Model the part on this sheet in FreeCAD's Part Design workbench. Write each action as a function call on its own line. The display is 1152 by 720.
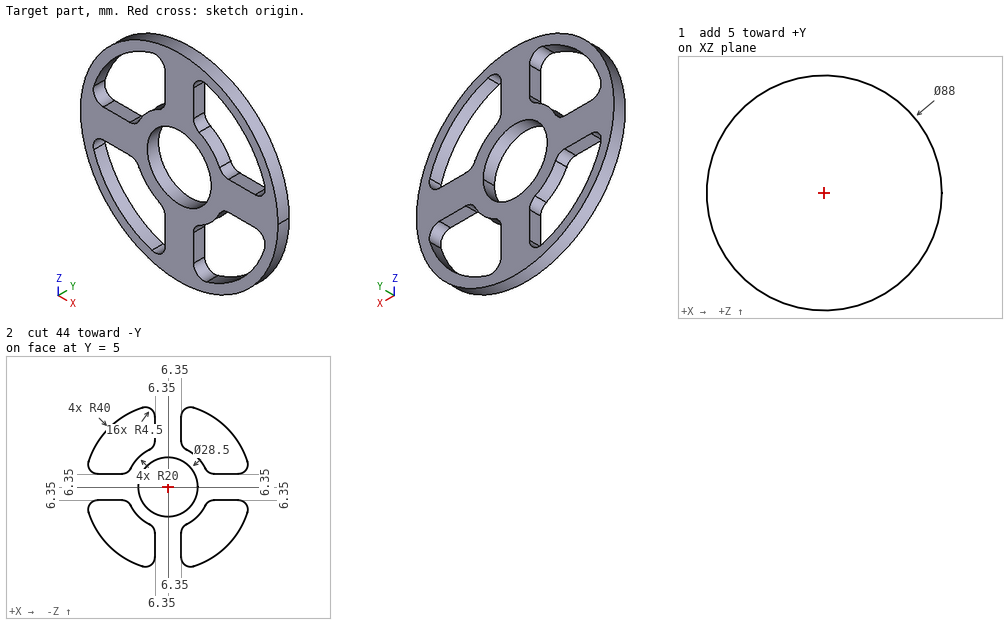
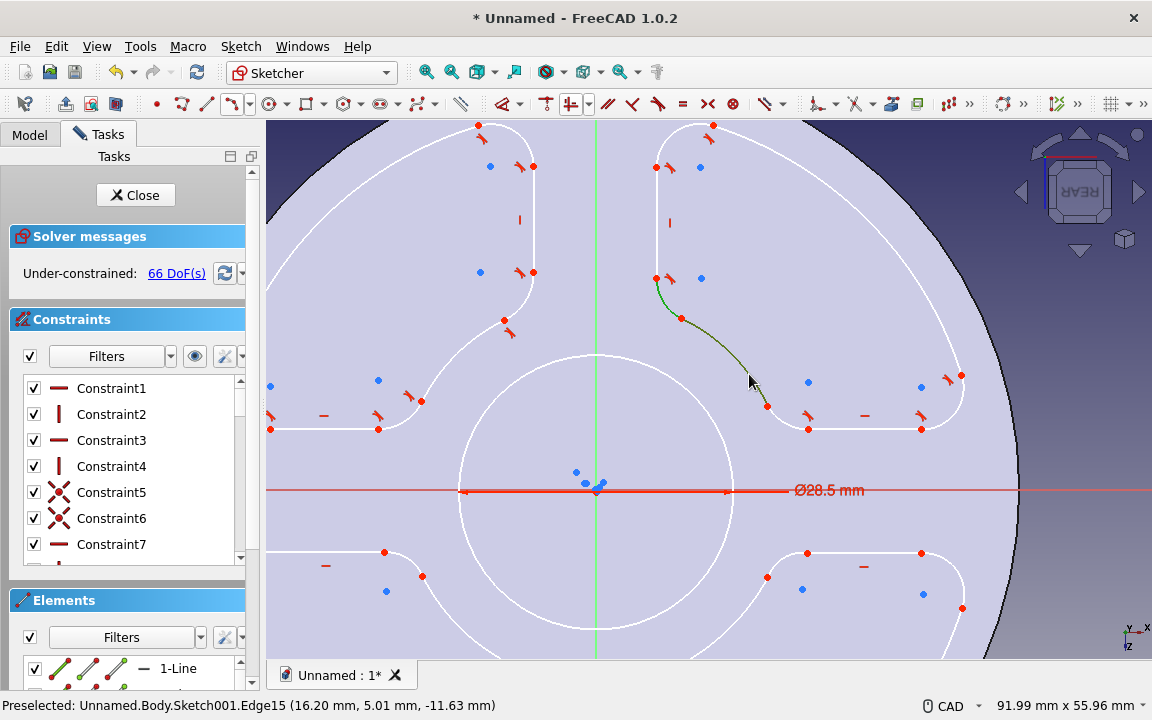
key(t)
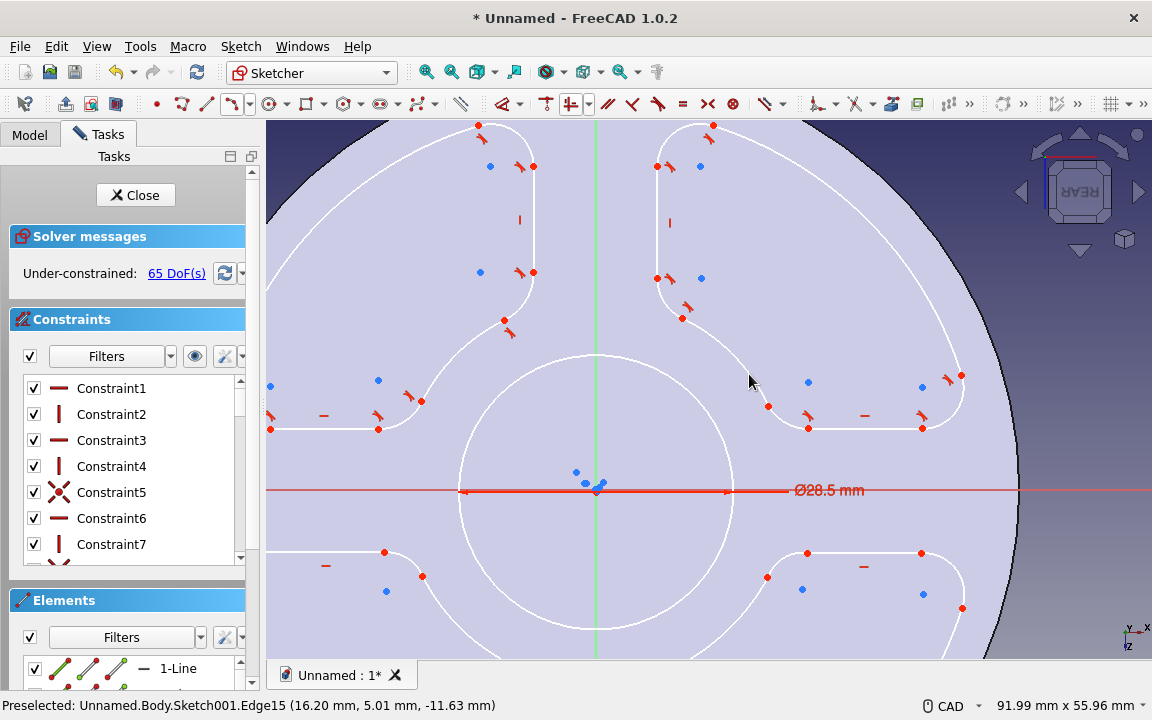
click(749, 374)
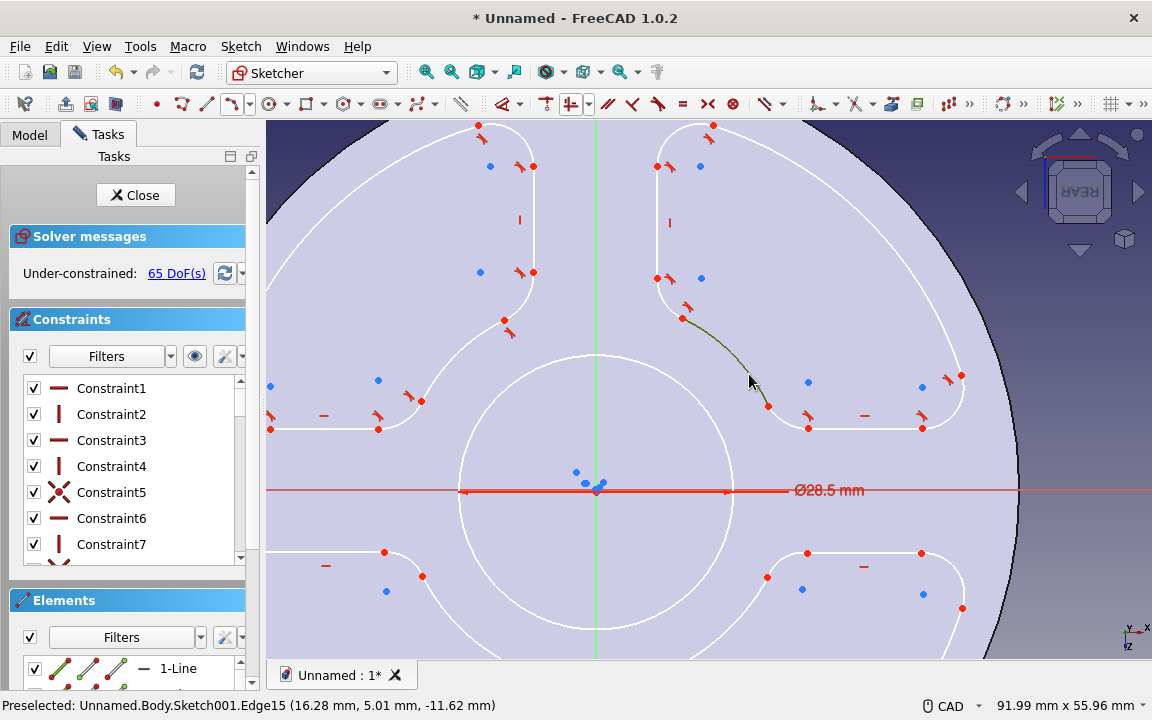
click(778, 417)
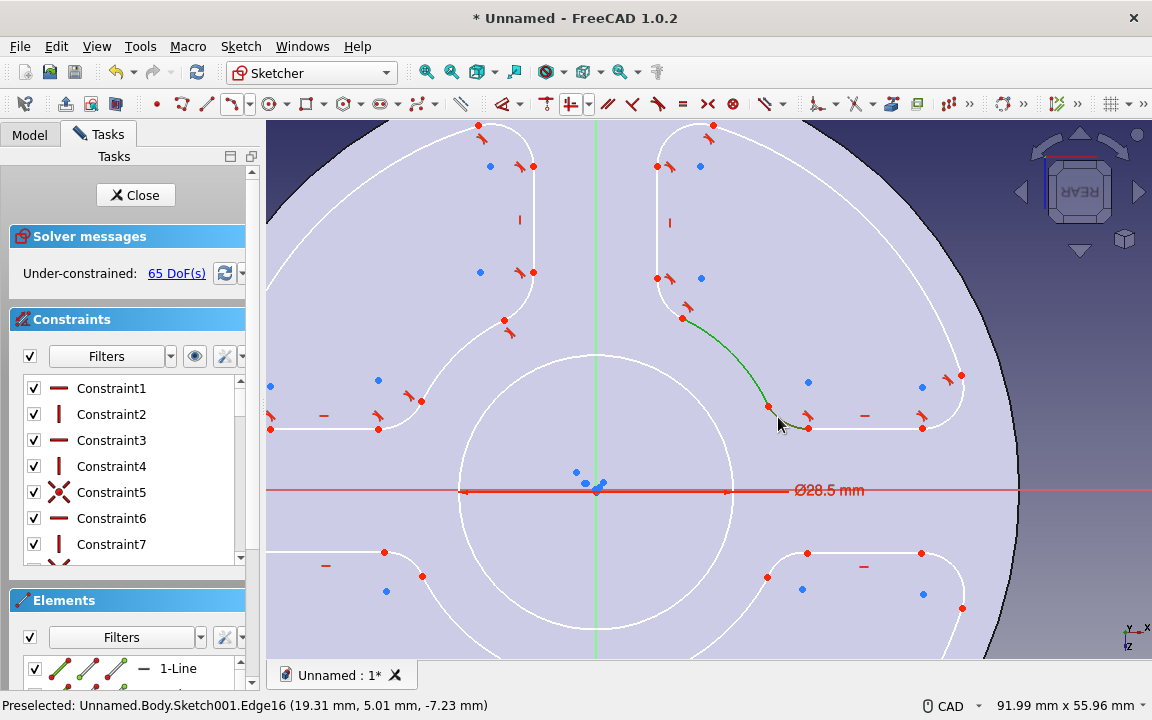
click(658, 104)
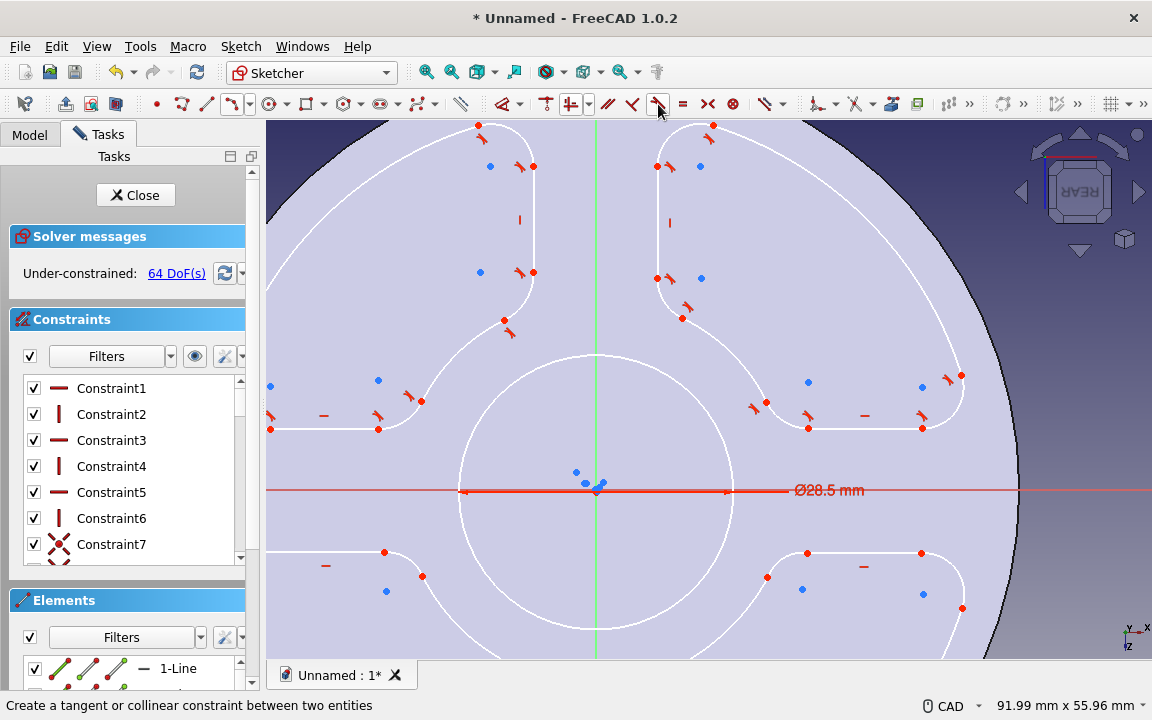
click(887, 553)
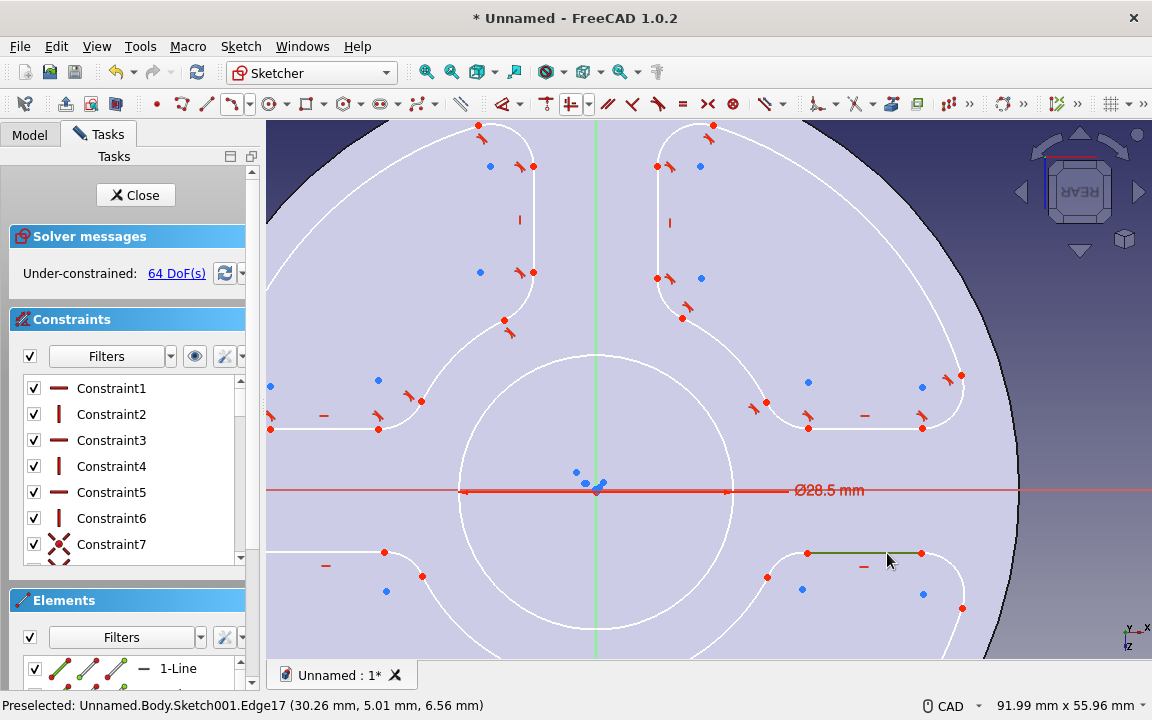
click(793, 554)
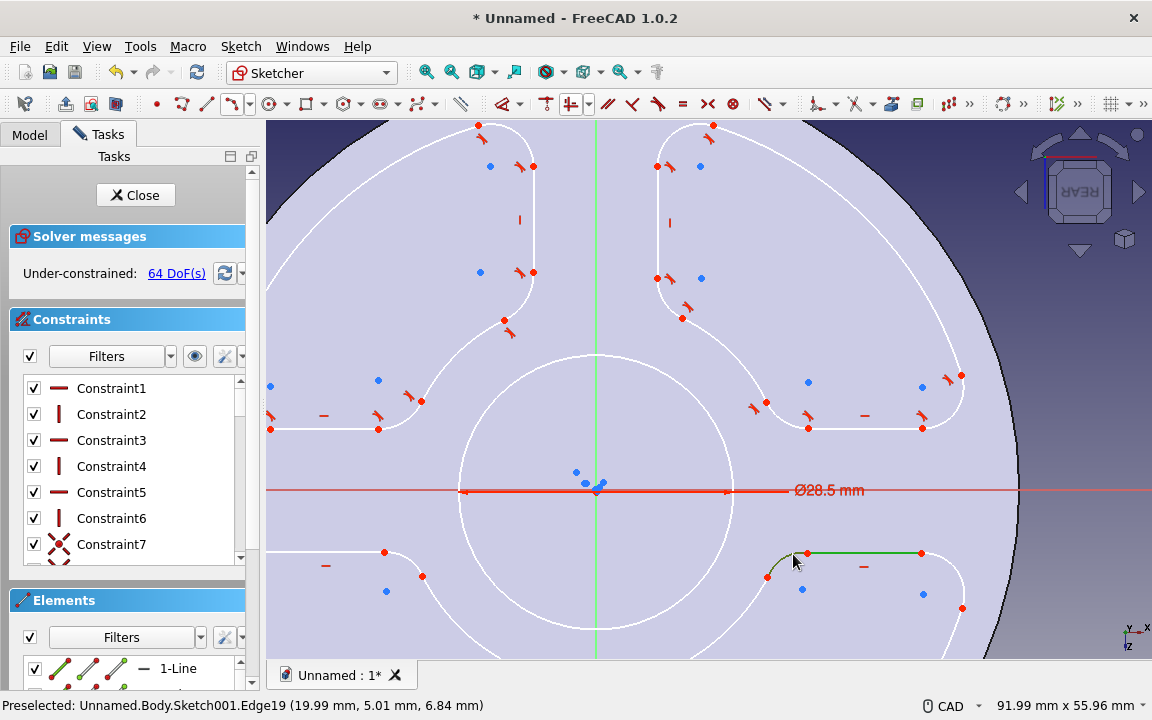
click(658, 104)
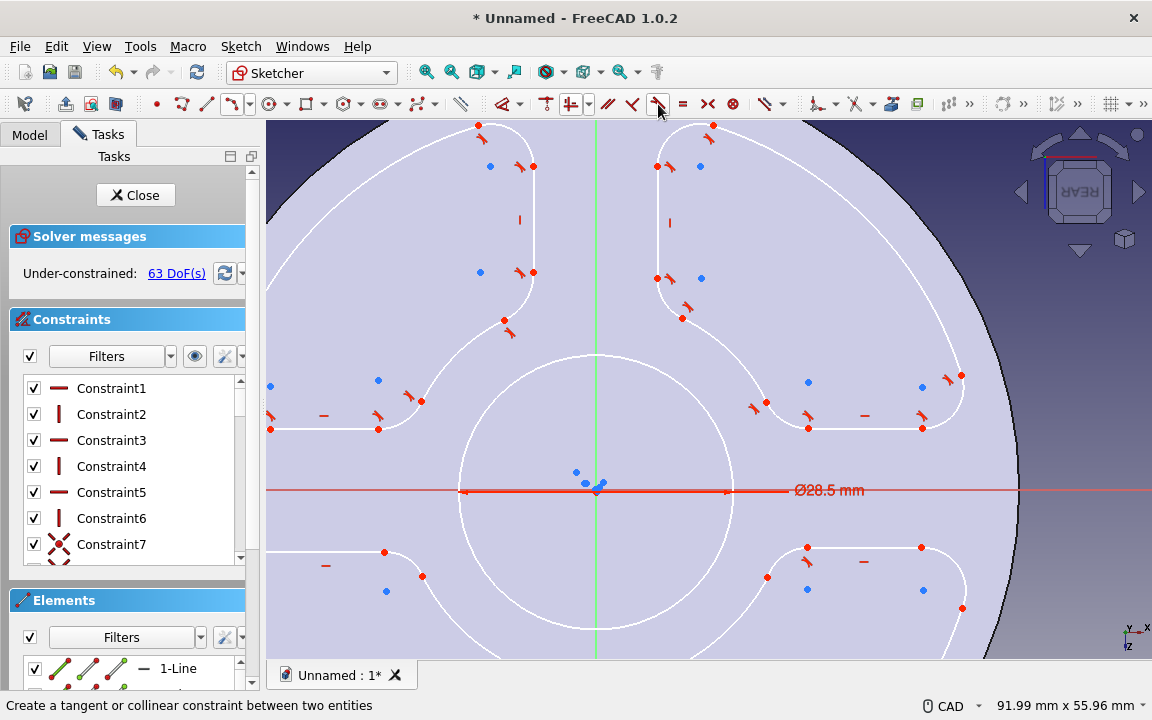
click(887, 548)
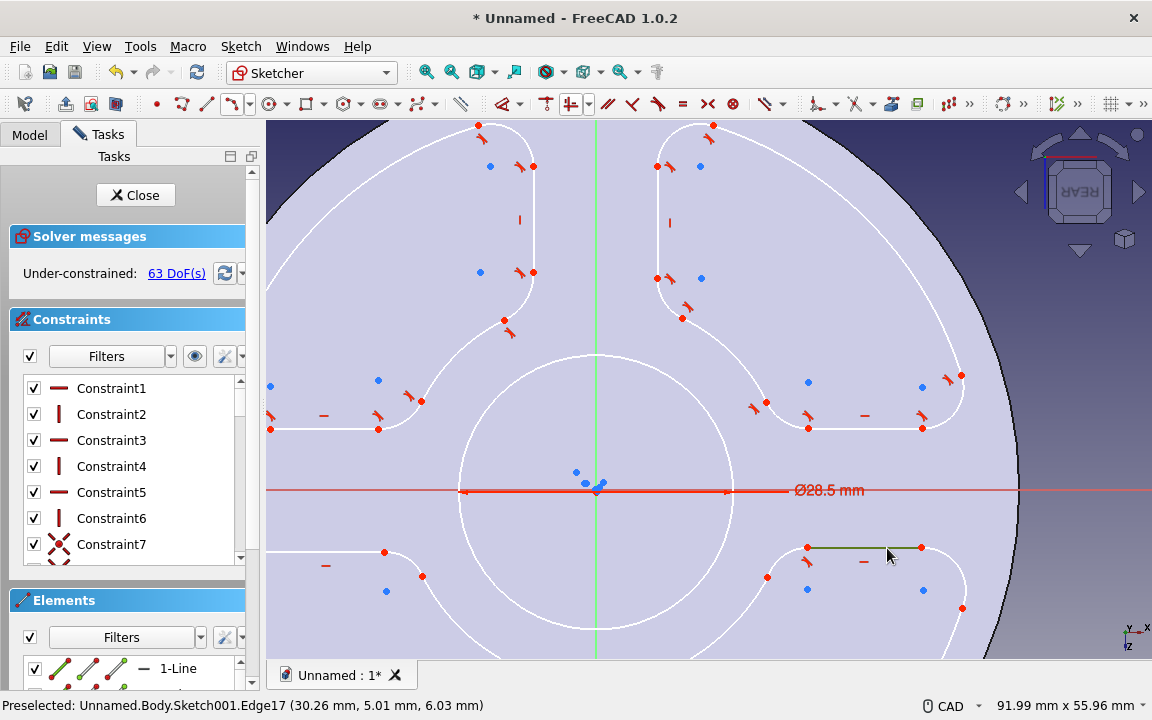
click(965, 583)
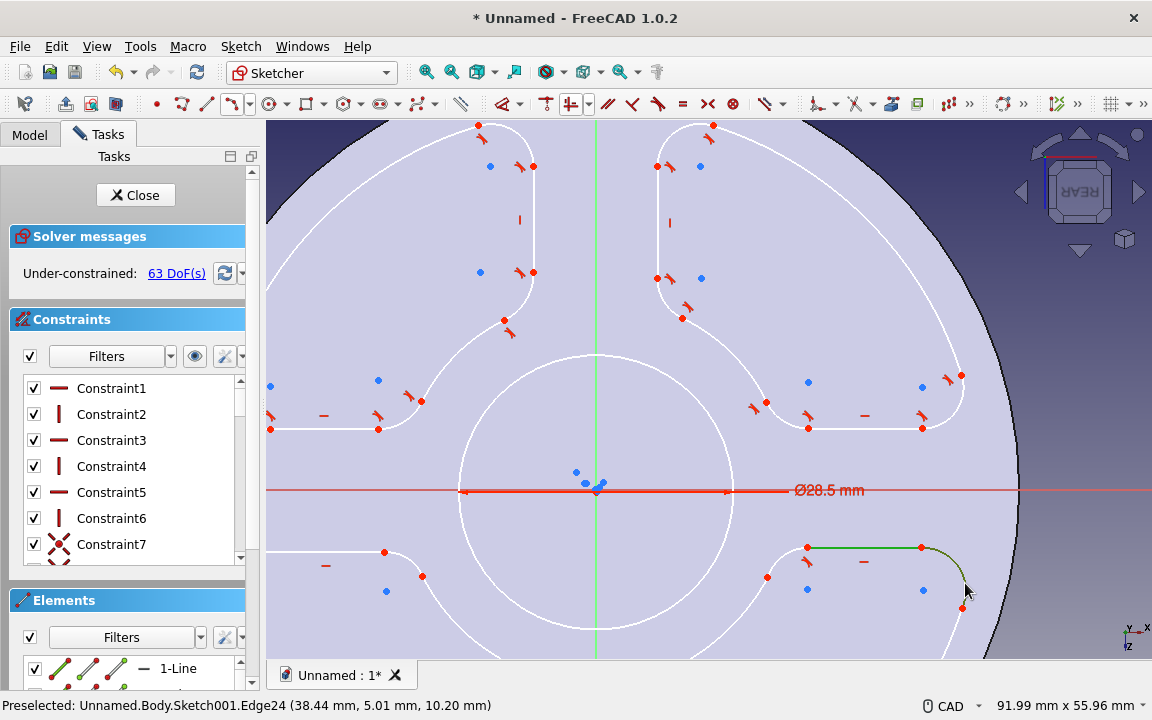
key(t)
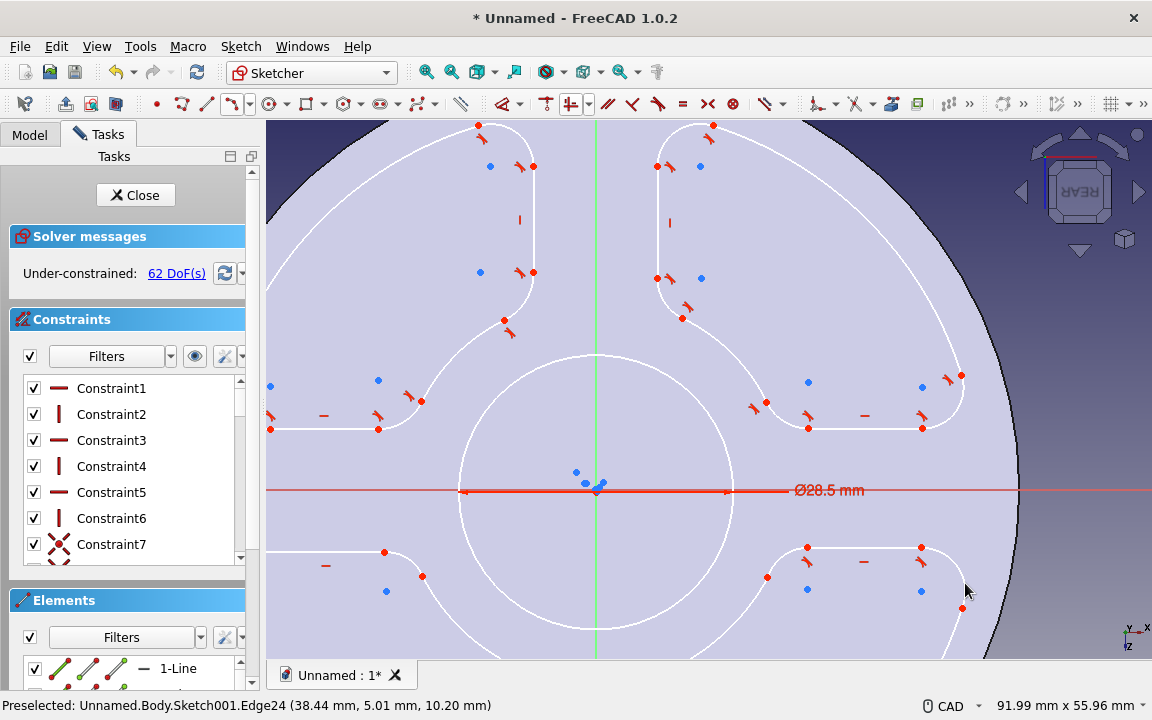
scroll(677, 308, down, 4)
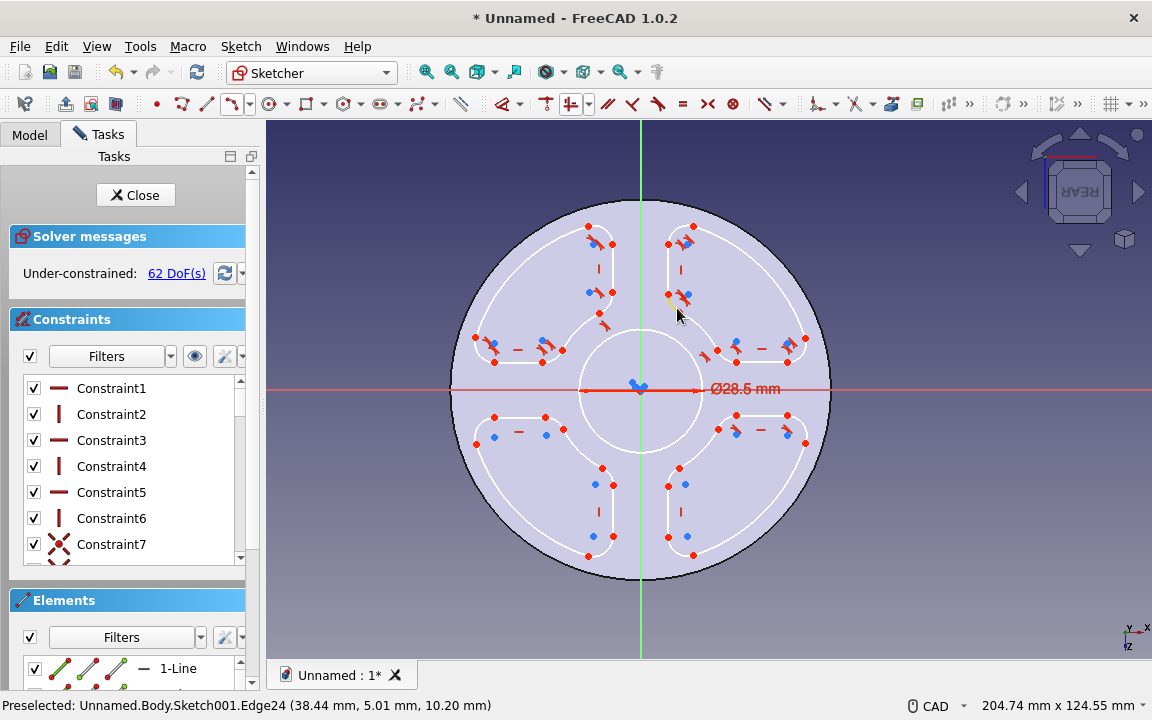
click(668, 502)